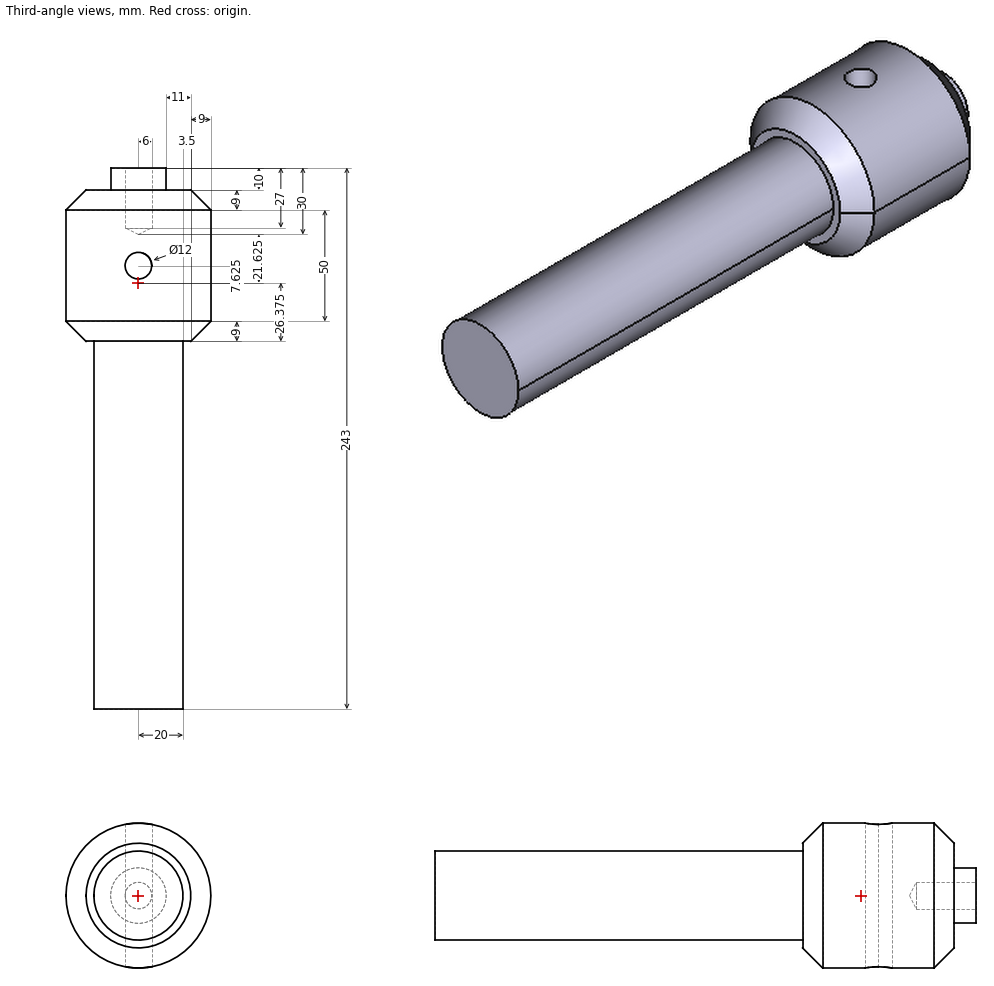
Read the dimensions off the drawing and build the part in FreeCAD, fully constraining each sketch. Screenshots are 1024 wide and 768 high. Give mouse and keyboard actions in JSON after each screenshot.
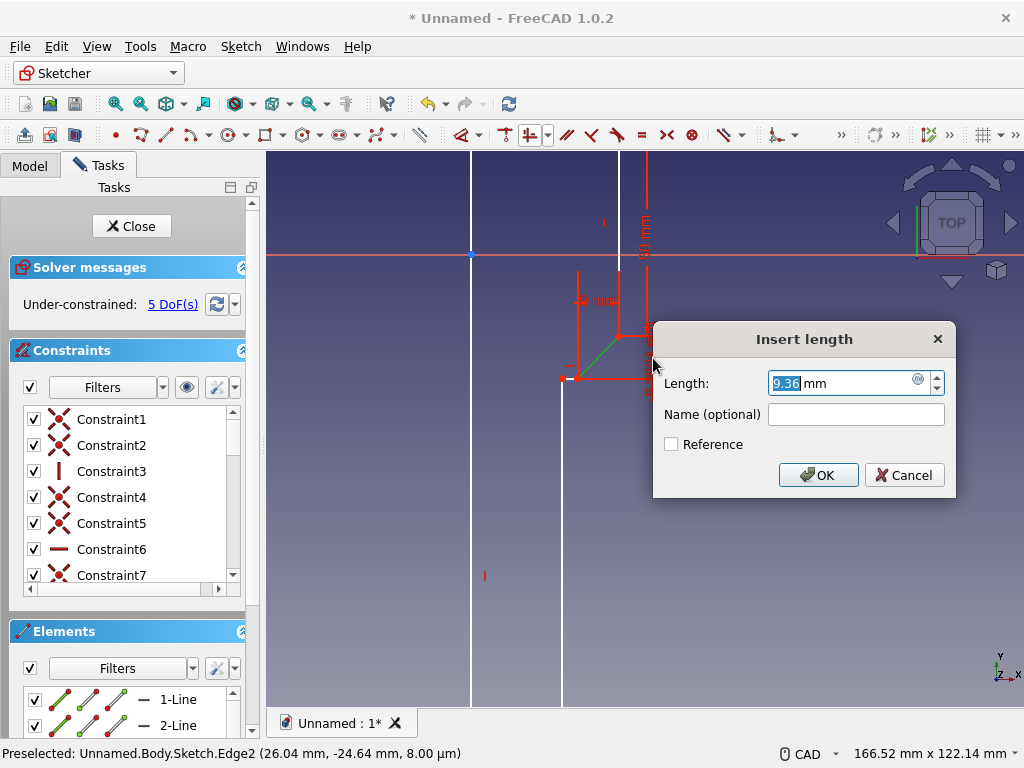
{"action": "type", "text": "9"}
{"action": "key", "text": "Return"}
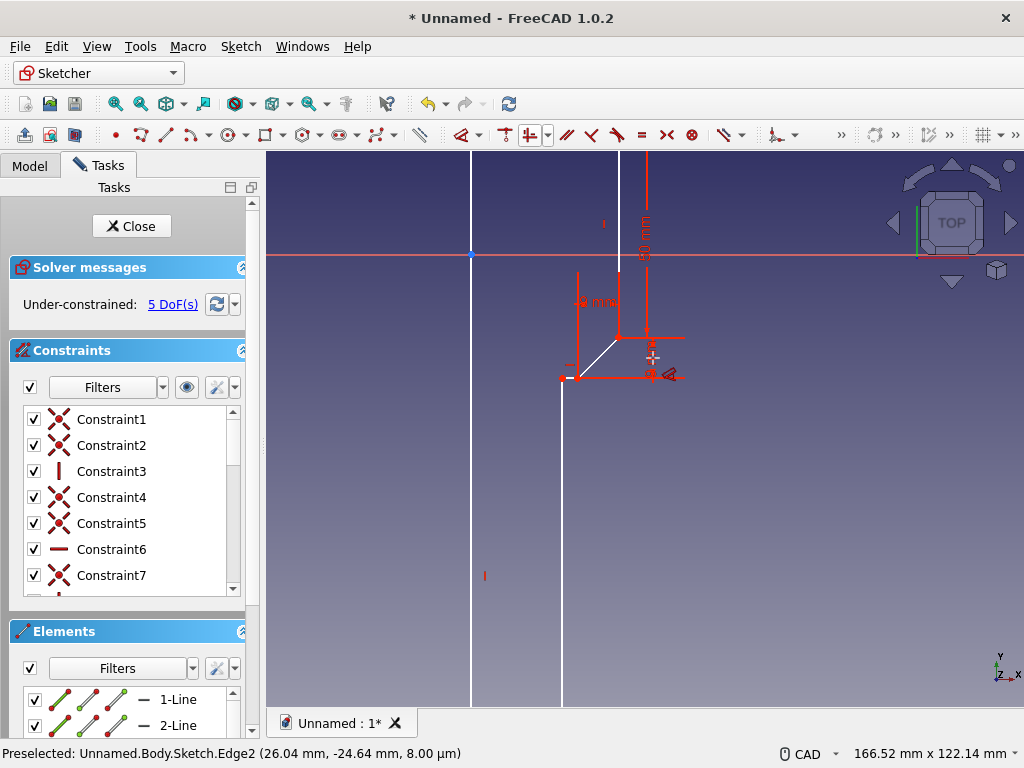
{"action": "scroll", "coordinate": [590, 367], "scroll_direction": "down", "scroll_amount": 6}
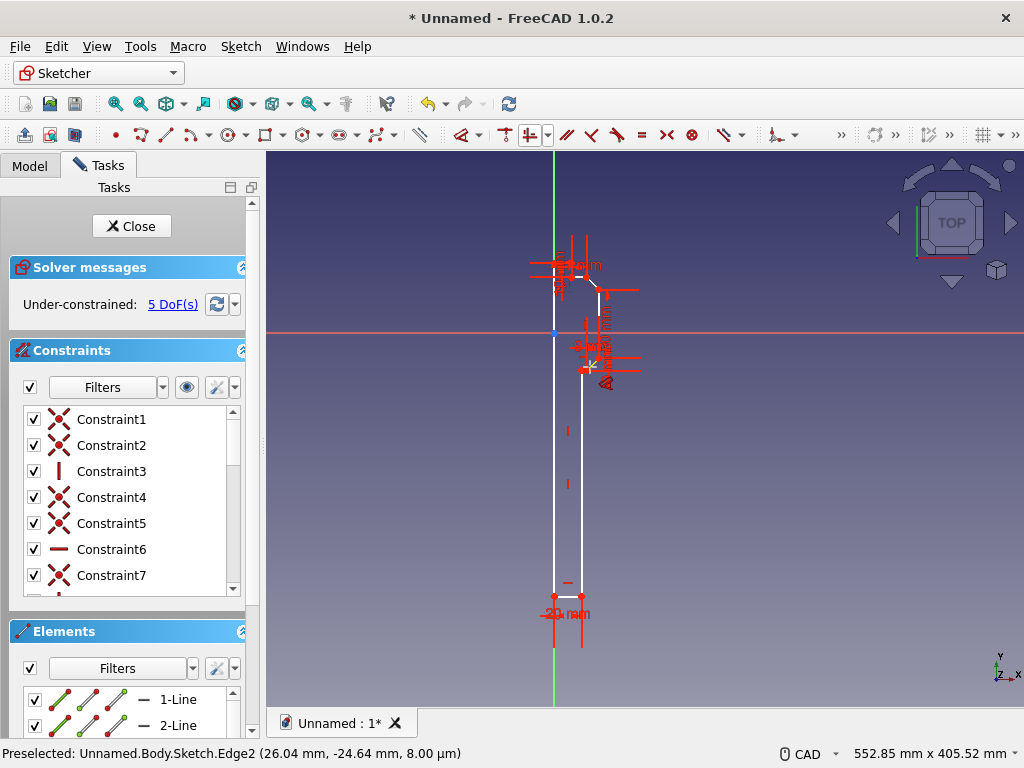
{"action": "scroll", "coordinate": [595, 286], "scroll_direction": "up", "scroll_amount": 6}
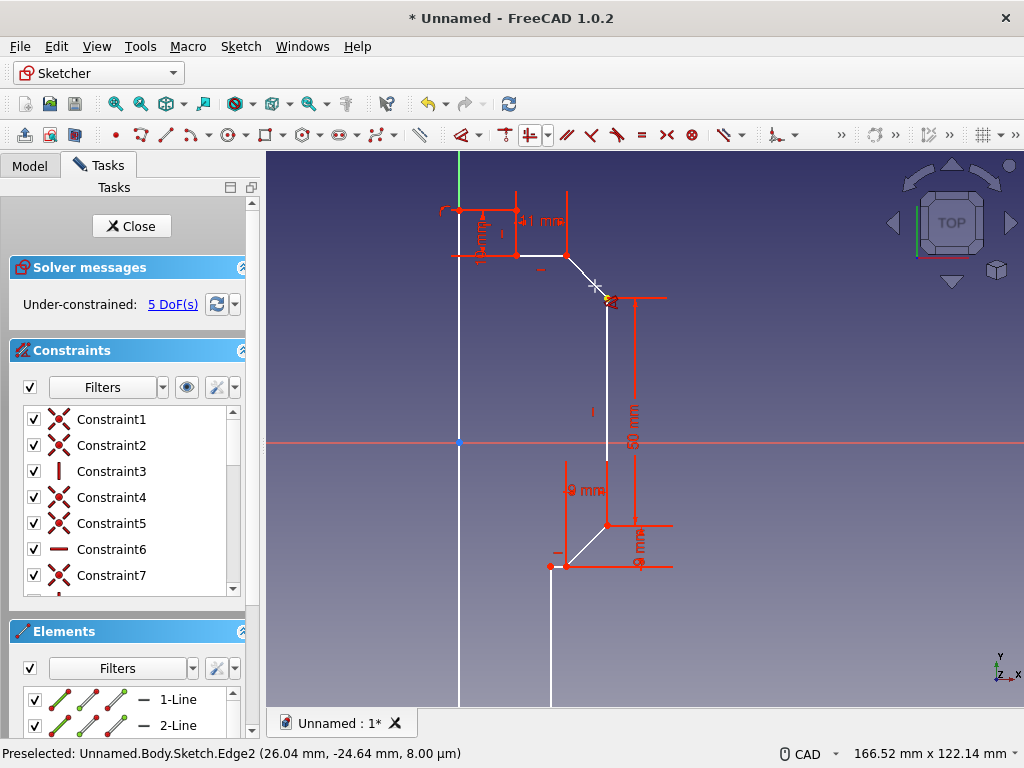
{"action": "left_click", "coordinate": [595, 285]}
{"action": "left_click", "coordinate": [587, 332]}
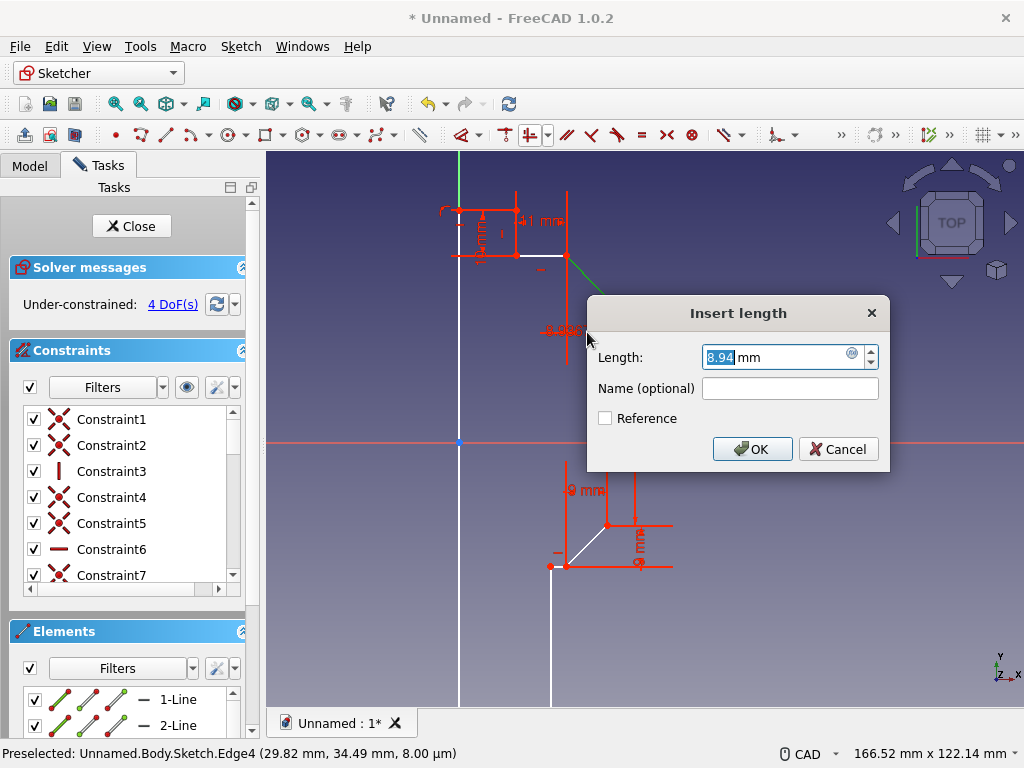
{"action": "type", "text": "9"}
{"action": "key", "text": "Return"}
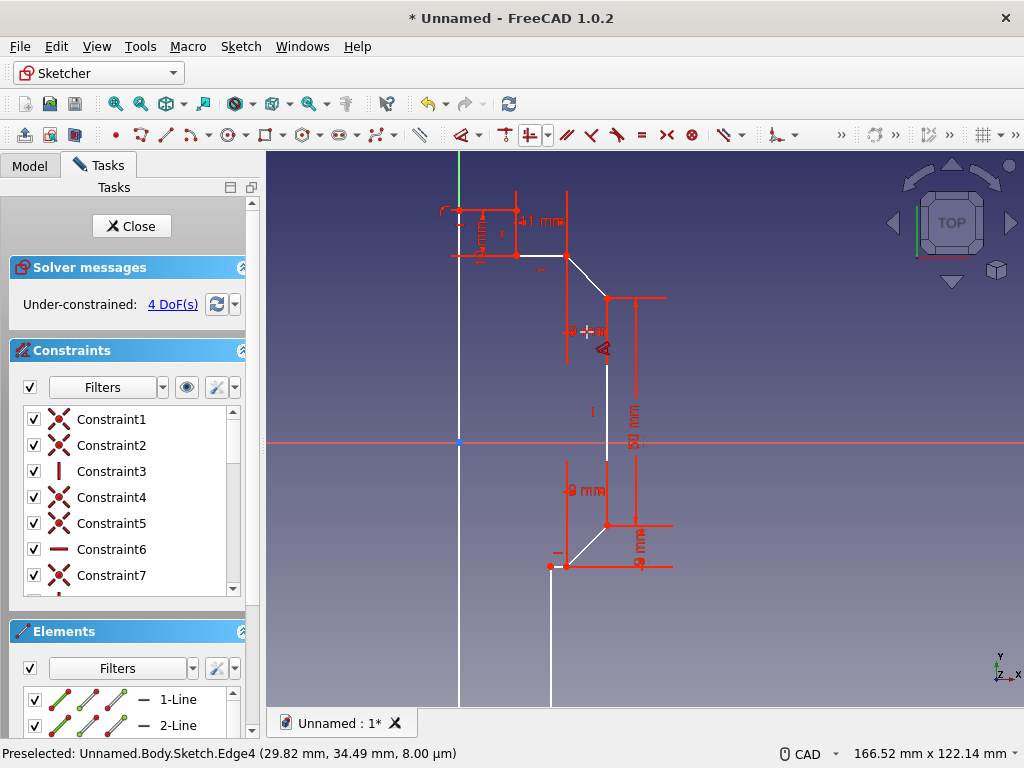
{"action": "left_click", "coordinate": [595, 285]}
{"action": "left_click", "coordinate": [641, 277]}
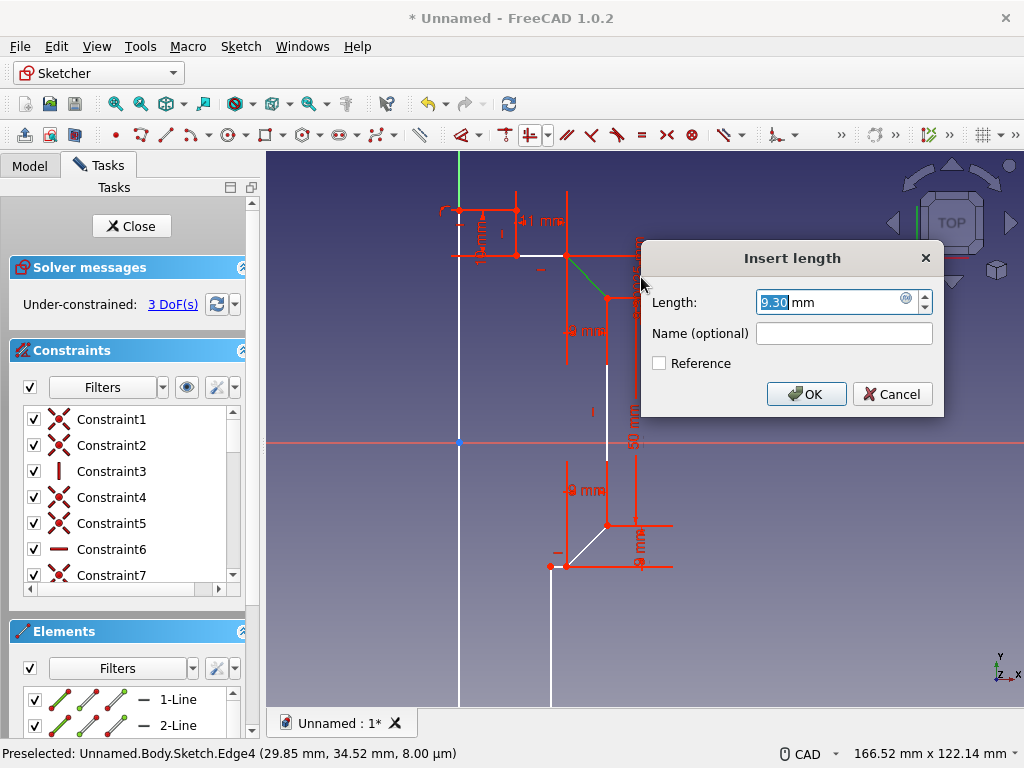
{"action": "type", "text": "9"}
{"action": "key", "text": "Return"}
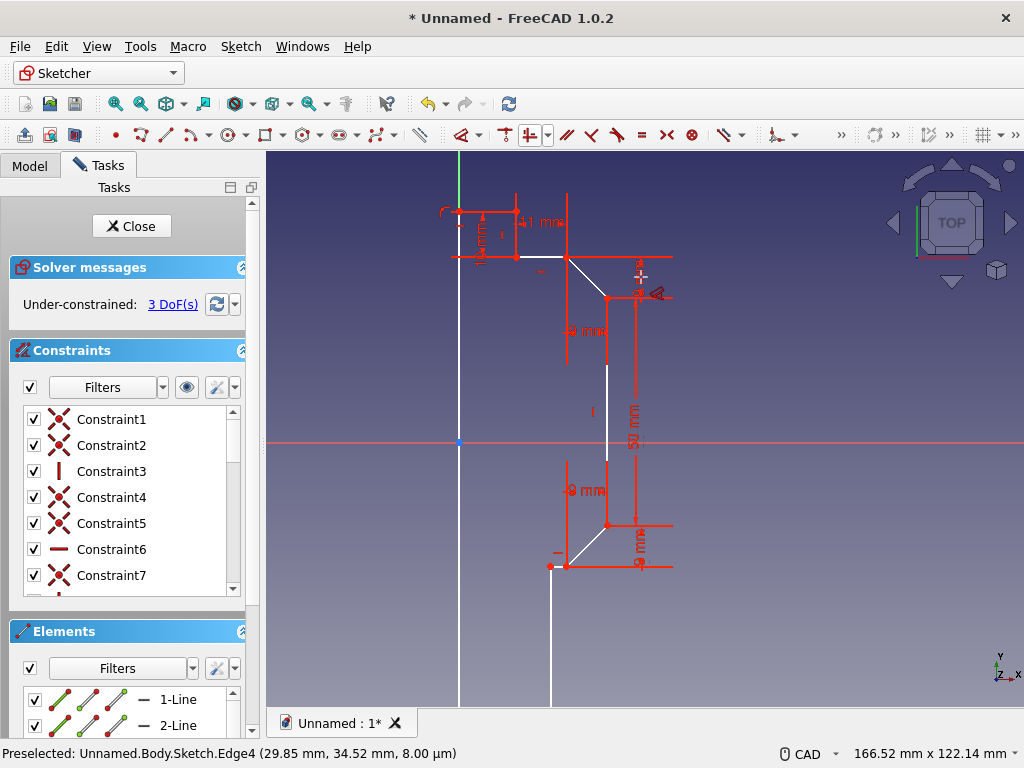
{"action": "scroll", "coordinate": [559, 567], "scroll_direction": "up", "scroll_amount": 5}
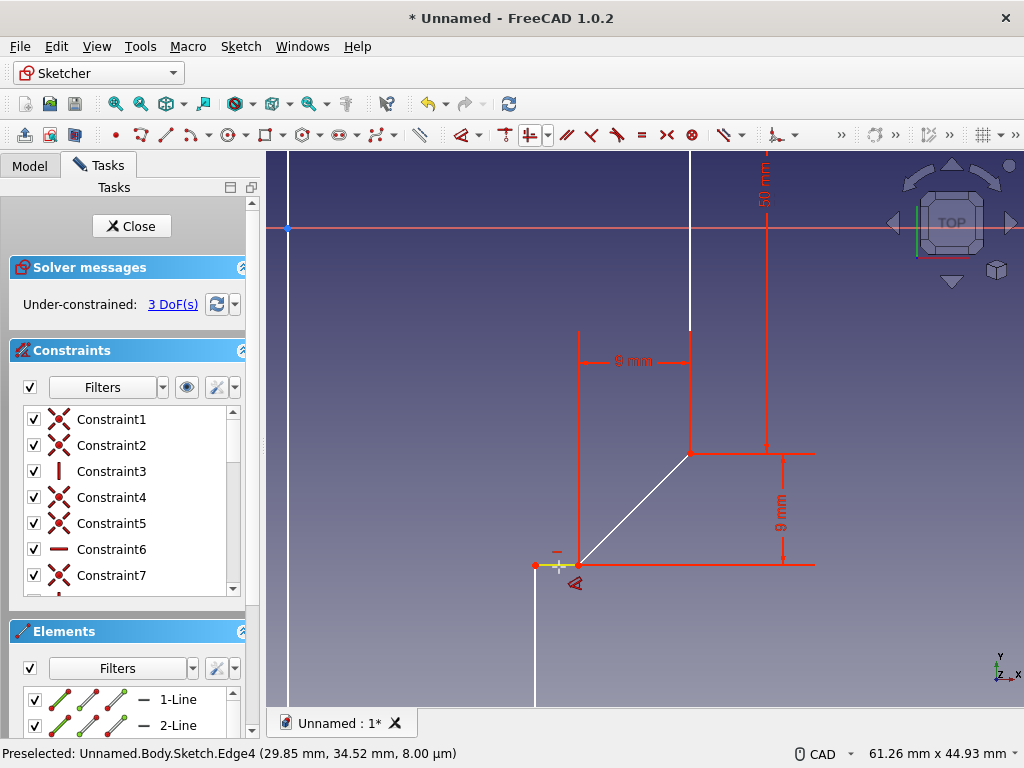
{"action": "left_click", "coordinate": [557, 565]}
{"action": "left_click", "coordinate": [557, 531]}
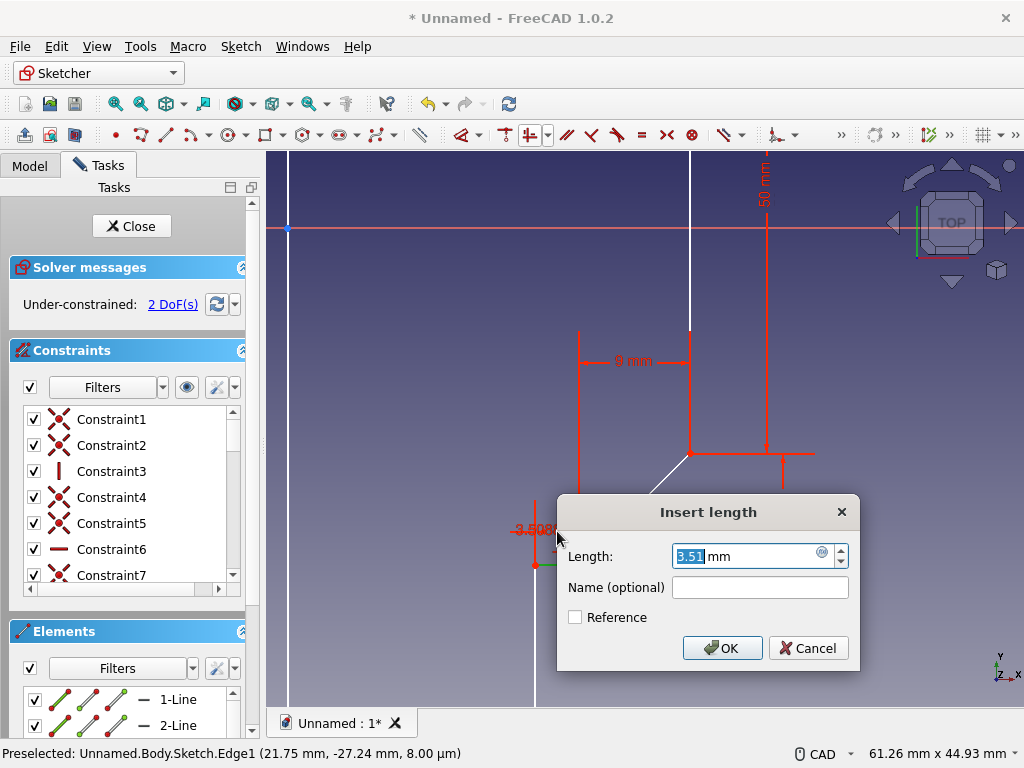
{"action": "type", "text": "3.5"}
{"action": "key", "text": "Return"}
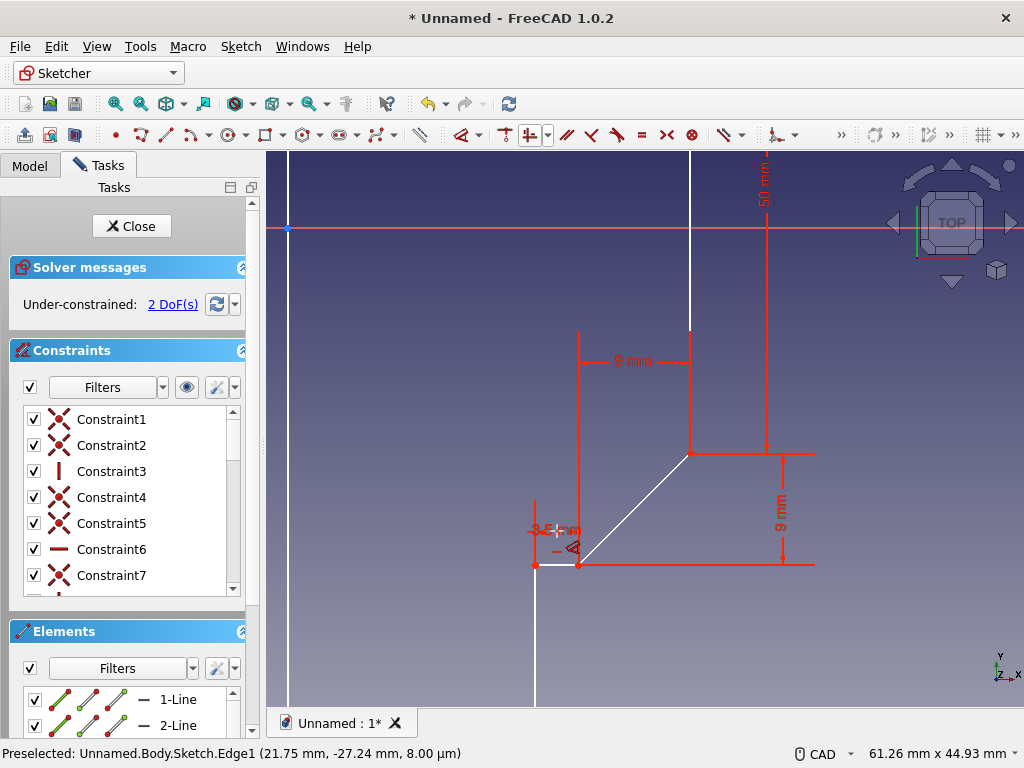
{"action": "scroll", "coordinate": [587, 346], "scroll_direction": "down", "scroll_amount": 11}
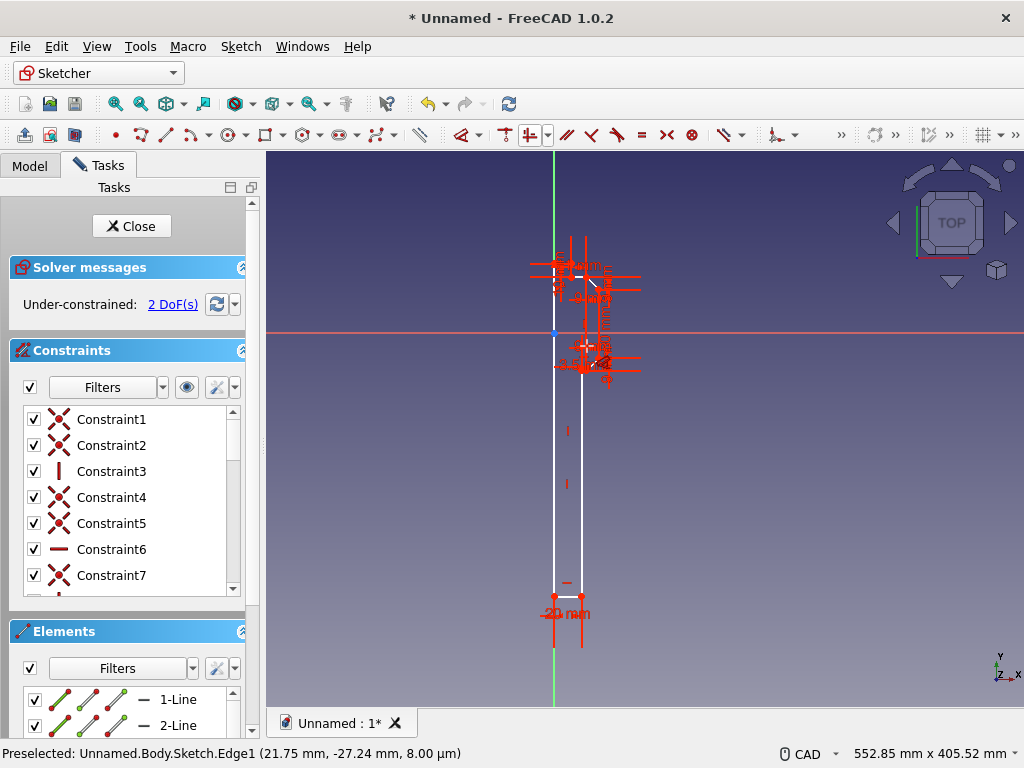
{"action": "left_click", "coordinate": [554, 364]}
{"action": "left_click", "coordinate": [520, 430]}